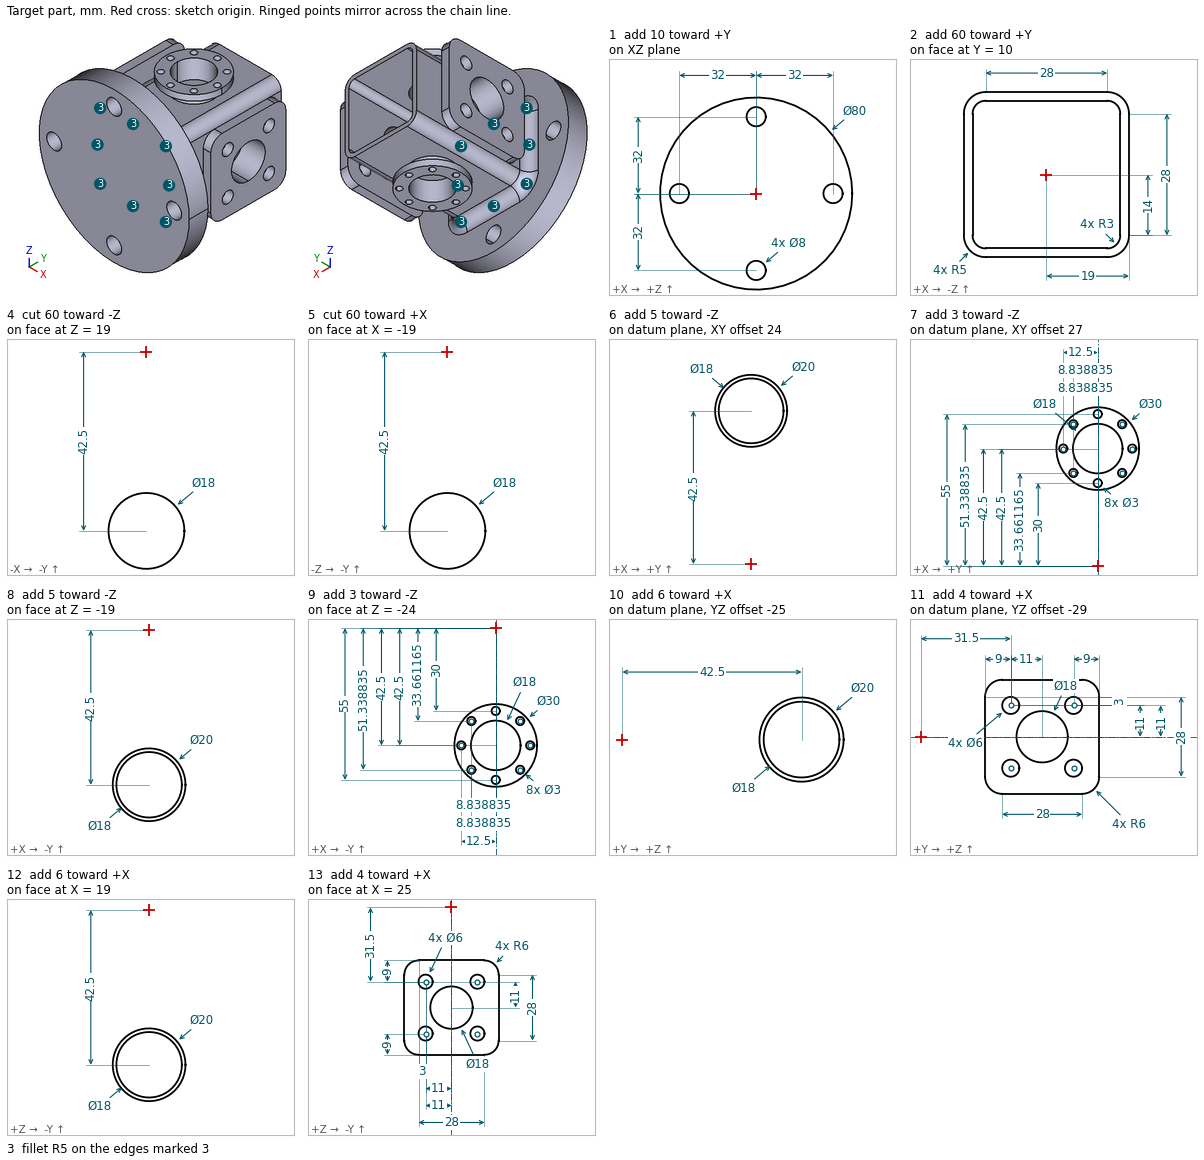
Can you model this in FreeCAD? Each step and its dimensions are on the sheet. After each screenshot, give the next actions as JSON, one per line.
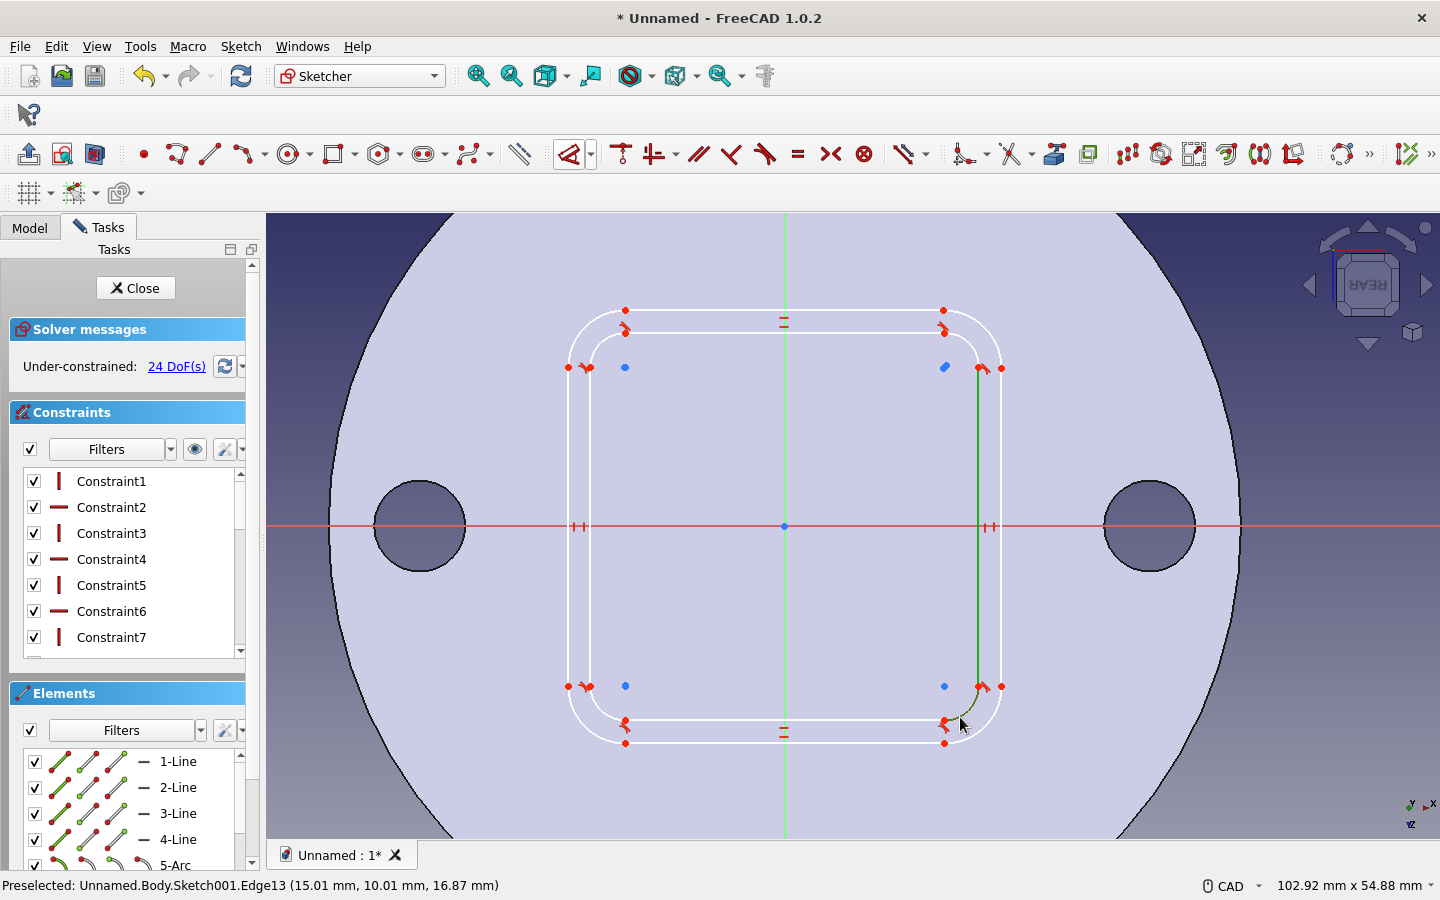
{"action": "key", "text": "t"}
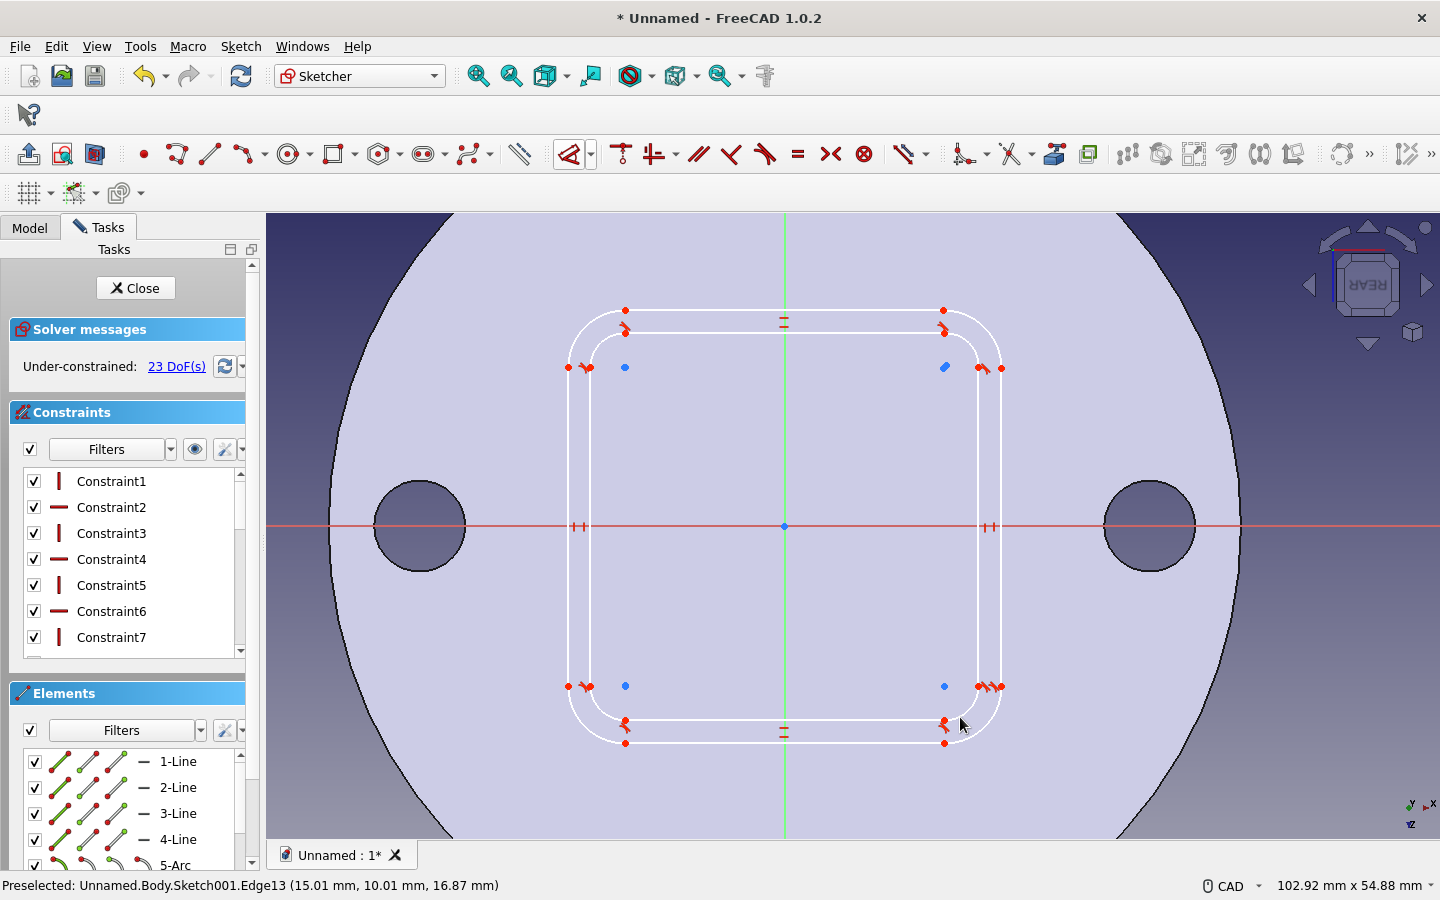
{"action": "left_click", "coordinate": [978, 463]}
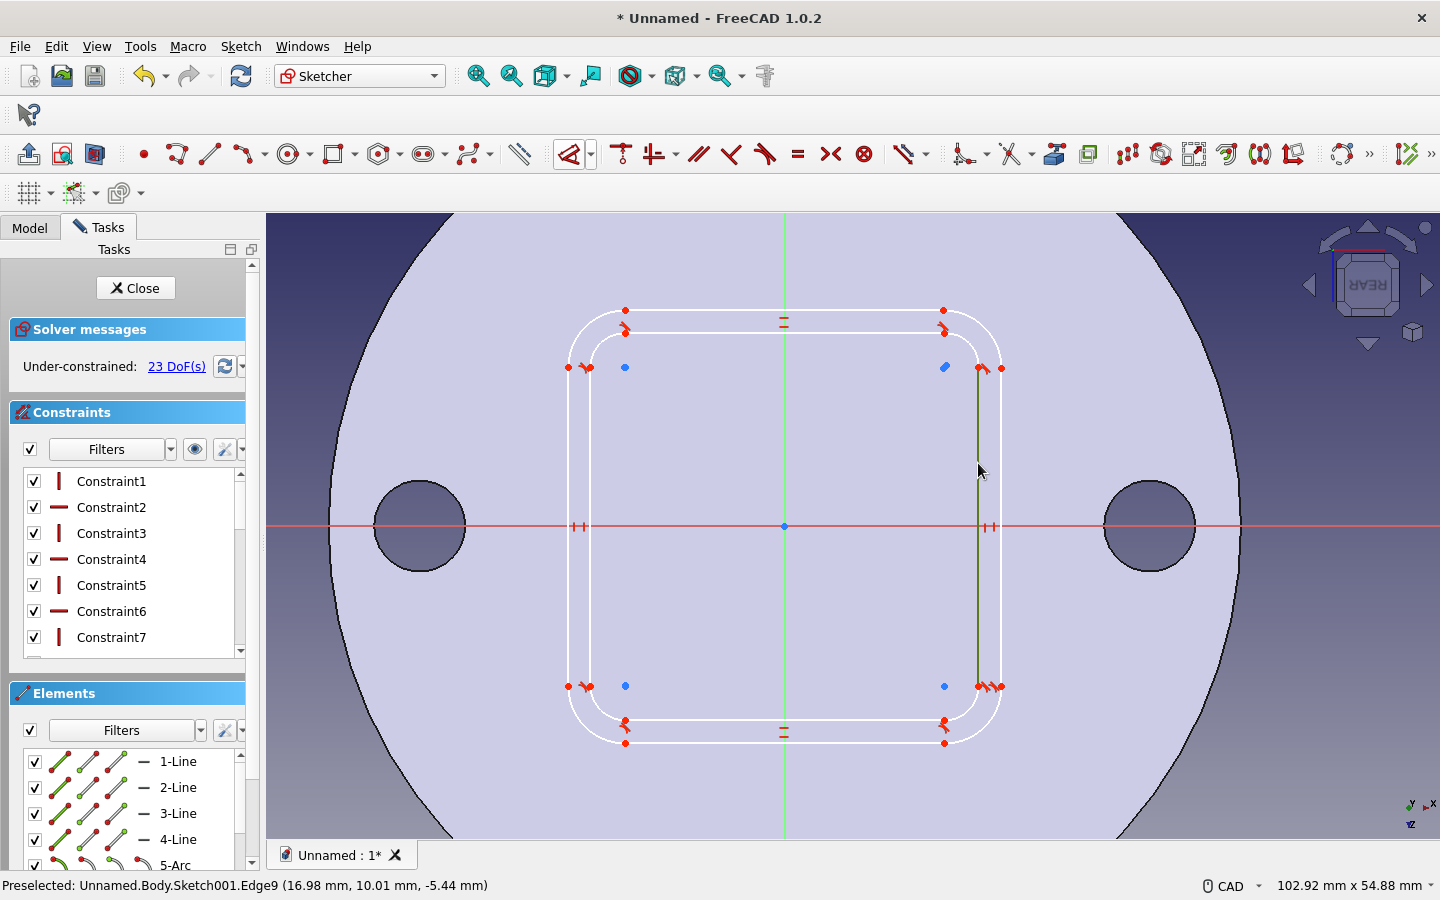
{"action": "left_click", "coordinate": [975, 352]}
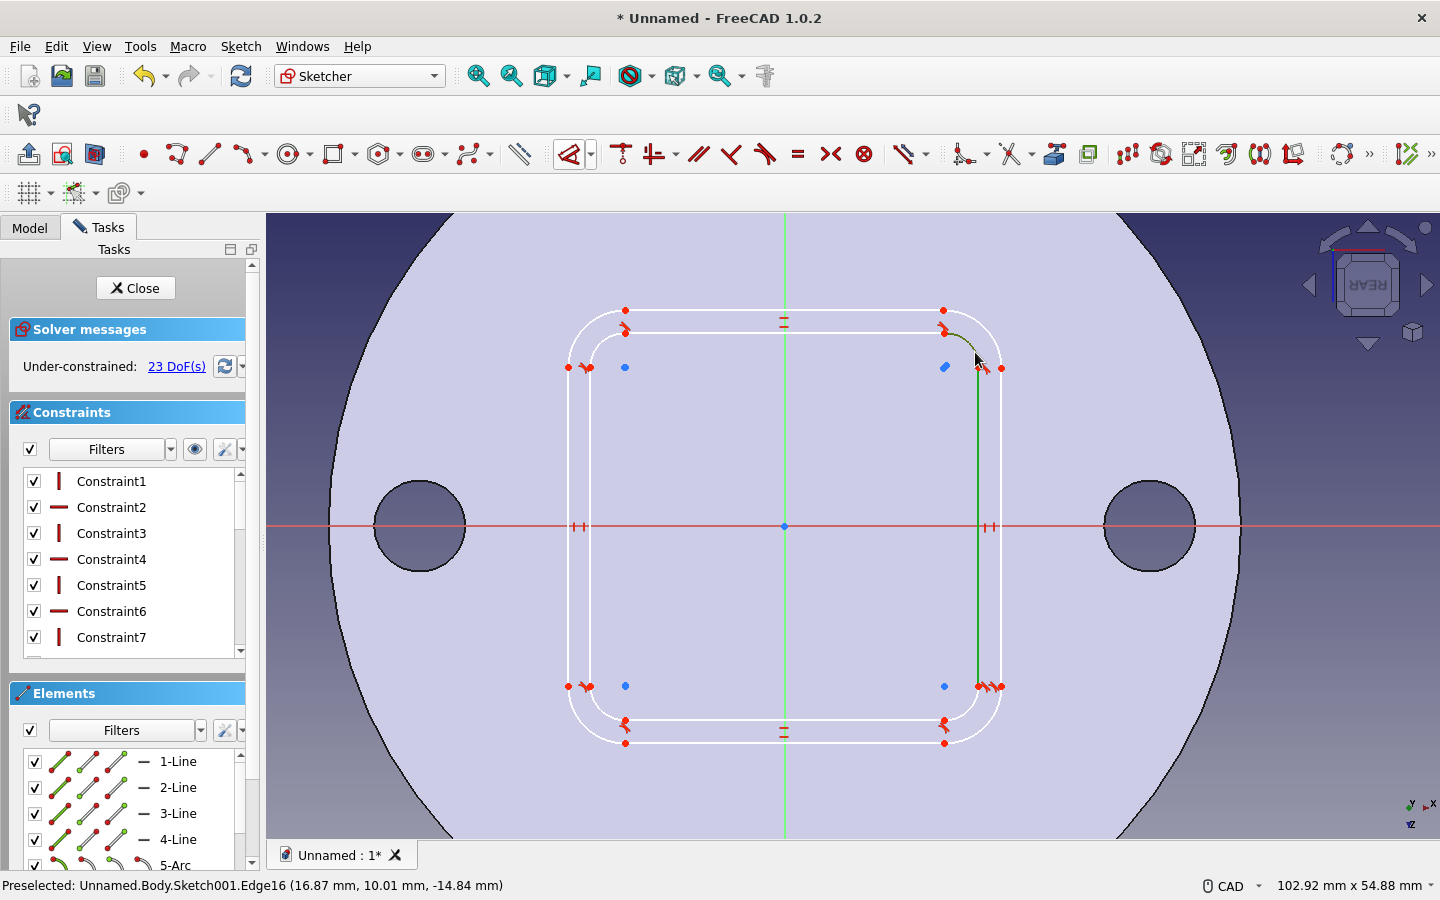
{"action": "left_click", "coordinate": [765, 154]}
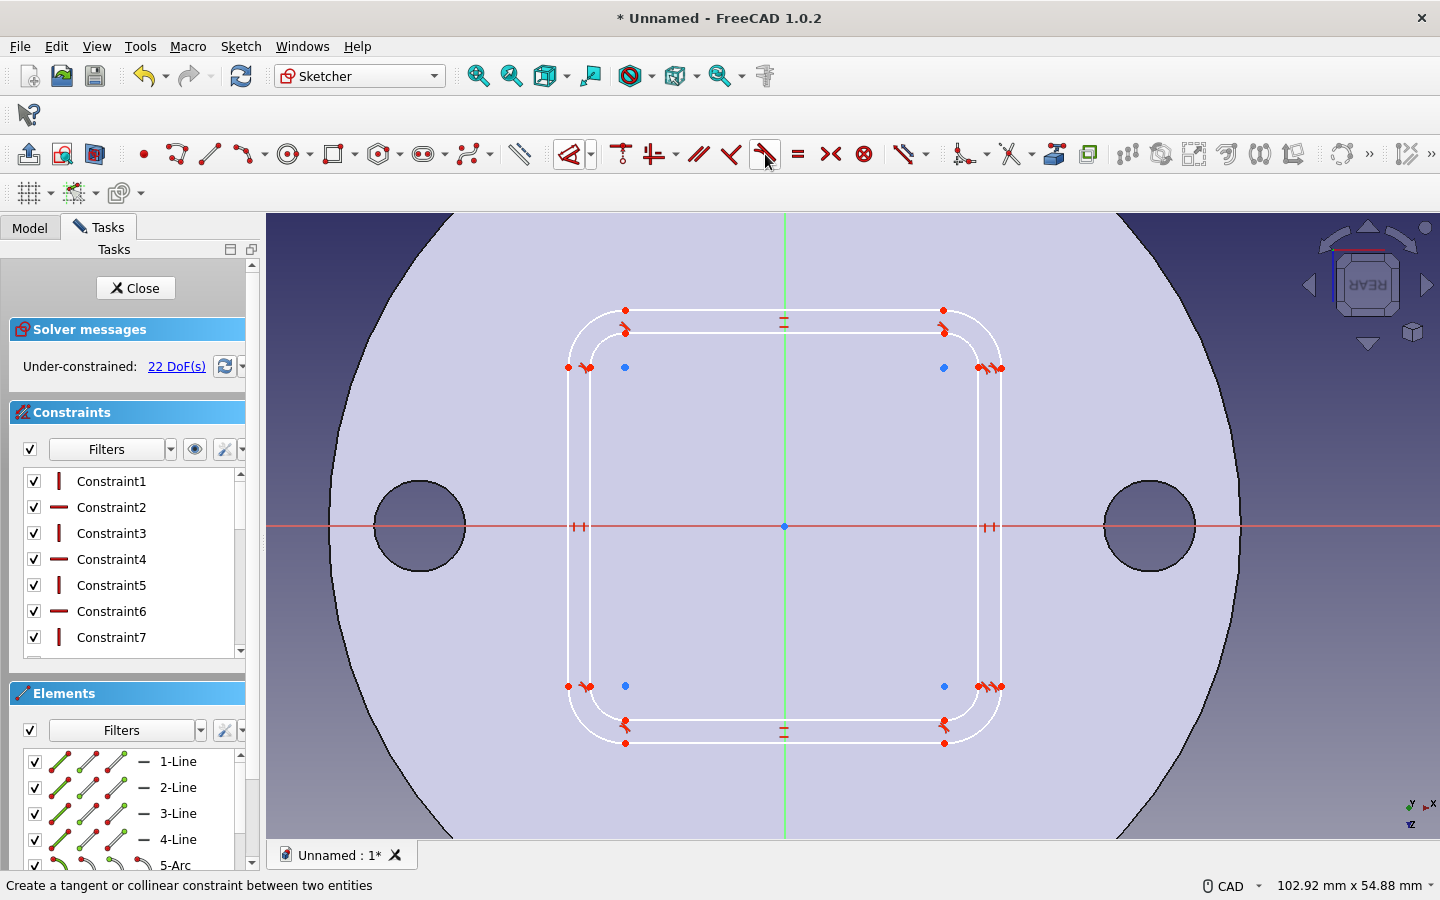
{"action": "left_click", "coordinate": [849, 720]}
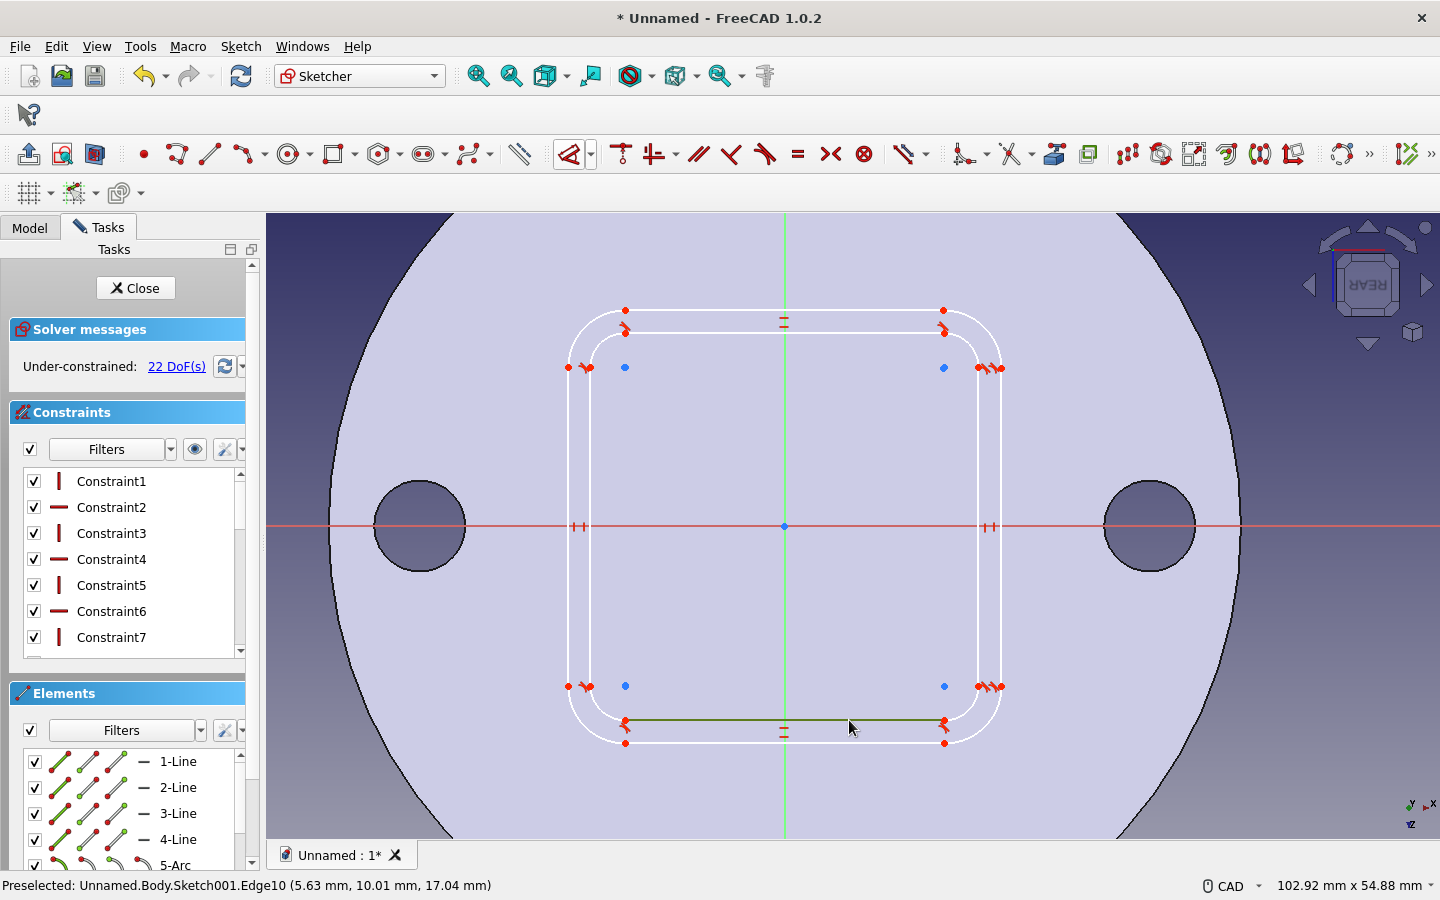
{"action": "left_click", "coordinate": [960, 717]}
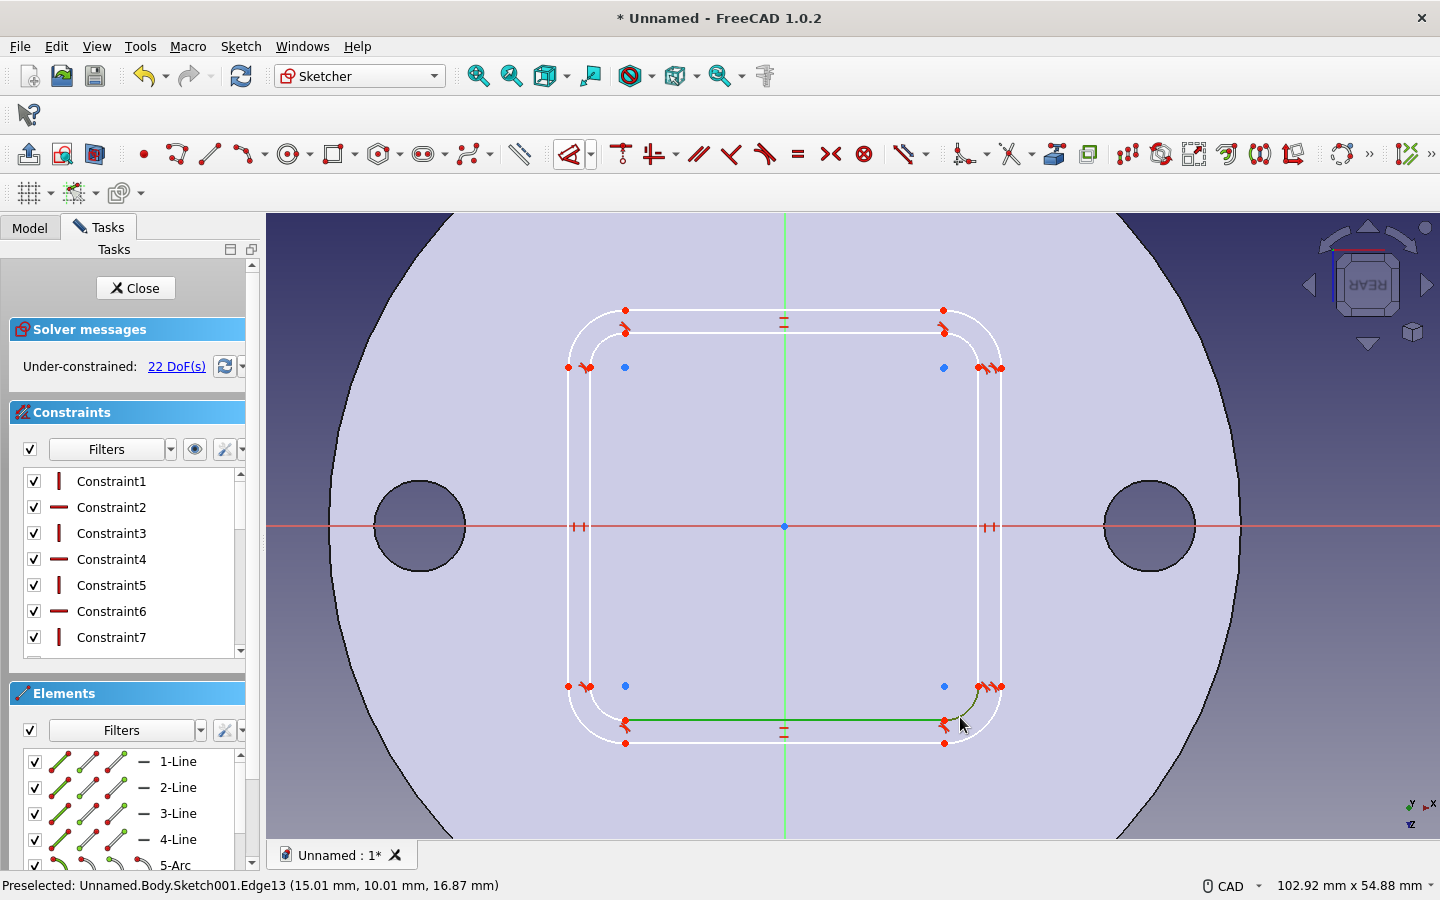
{"action": "key", "text": "t"}